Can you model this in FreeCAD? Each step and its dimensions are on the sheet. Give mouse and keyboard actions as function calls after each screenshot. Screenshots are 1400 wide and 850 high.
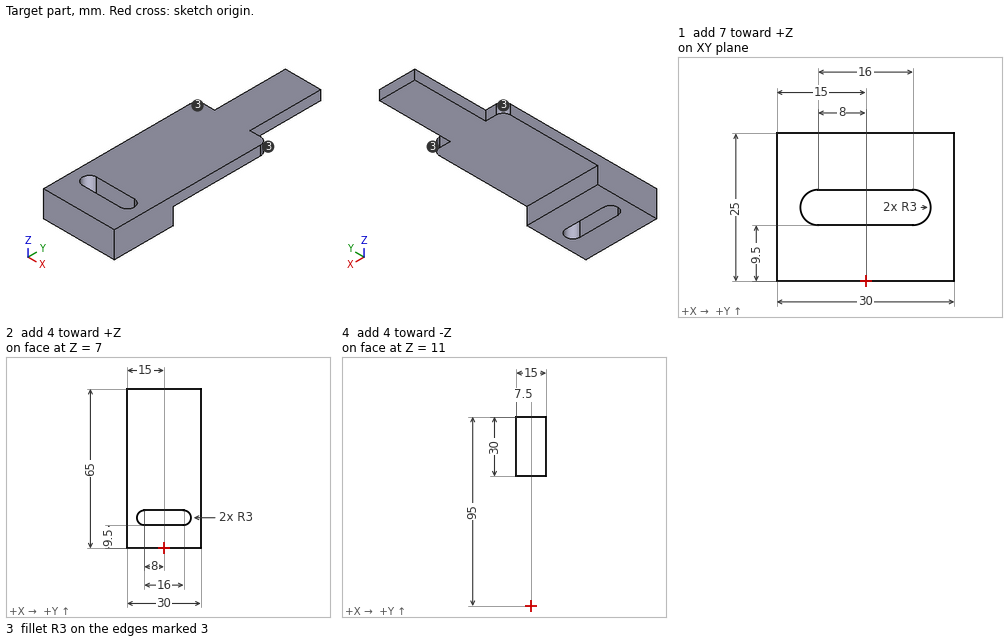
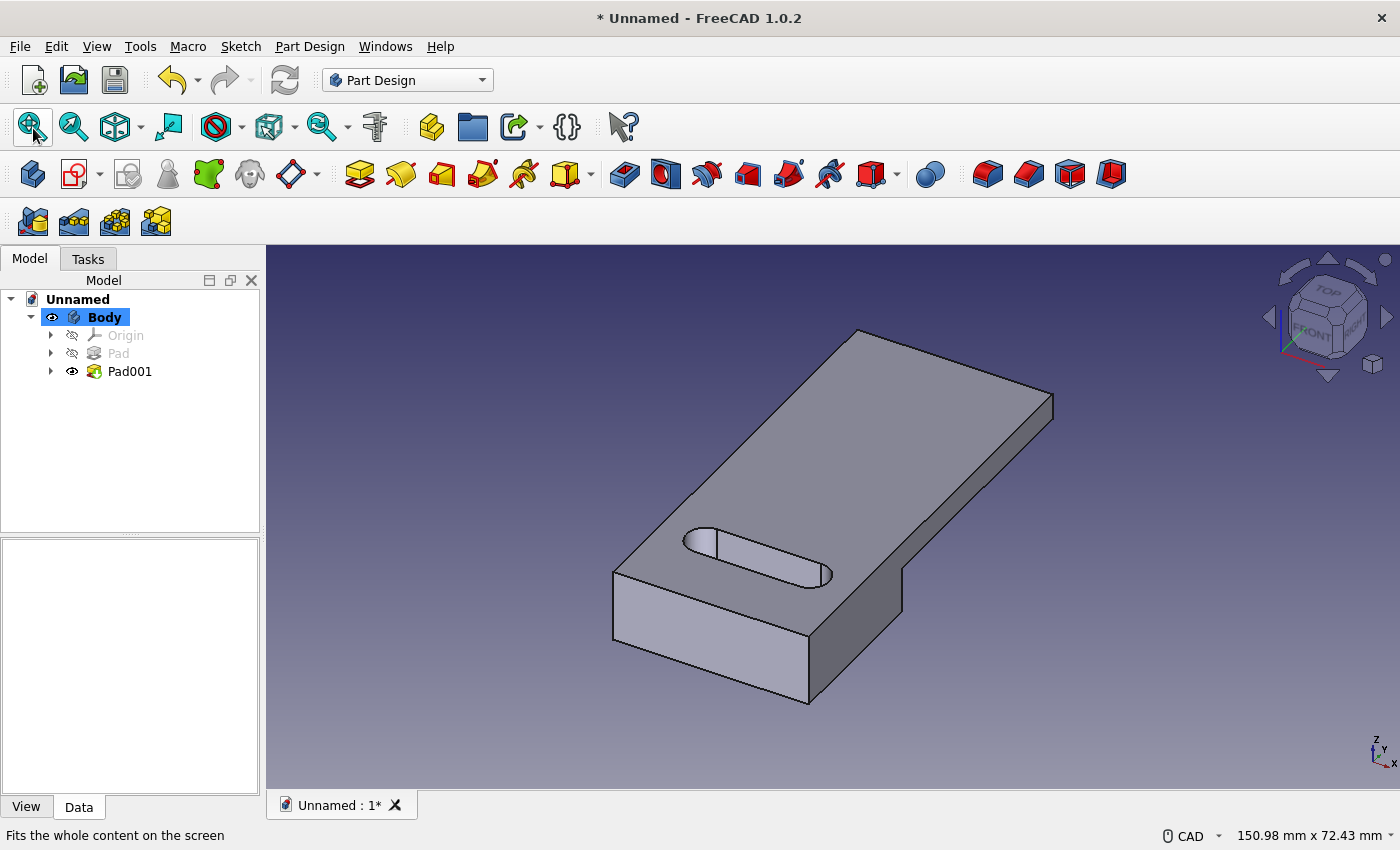
key(0)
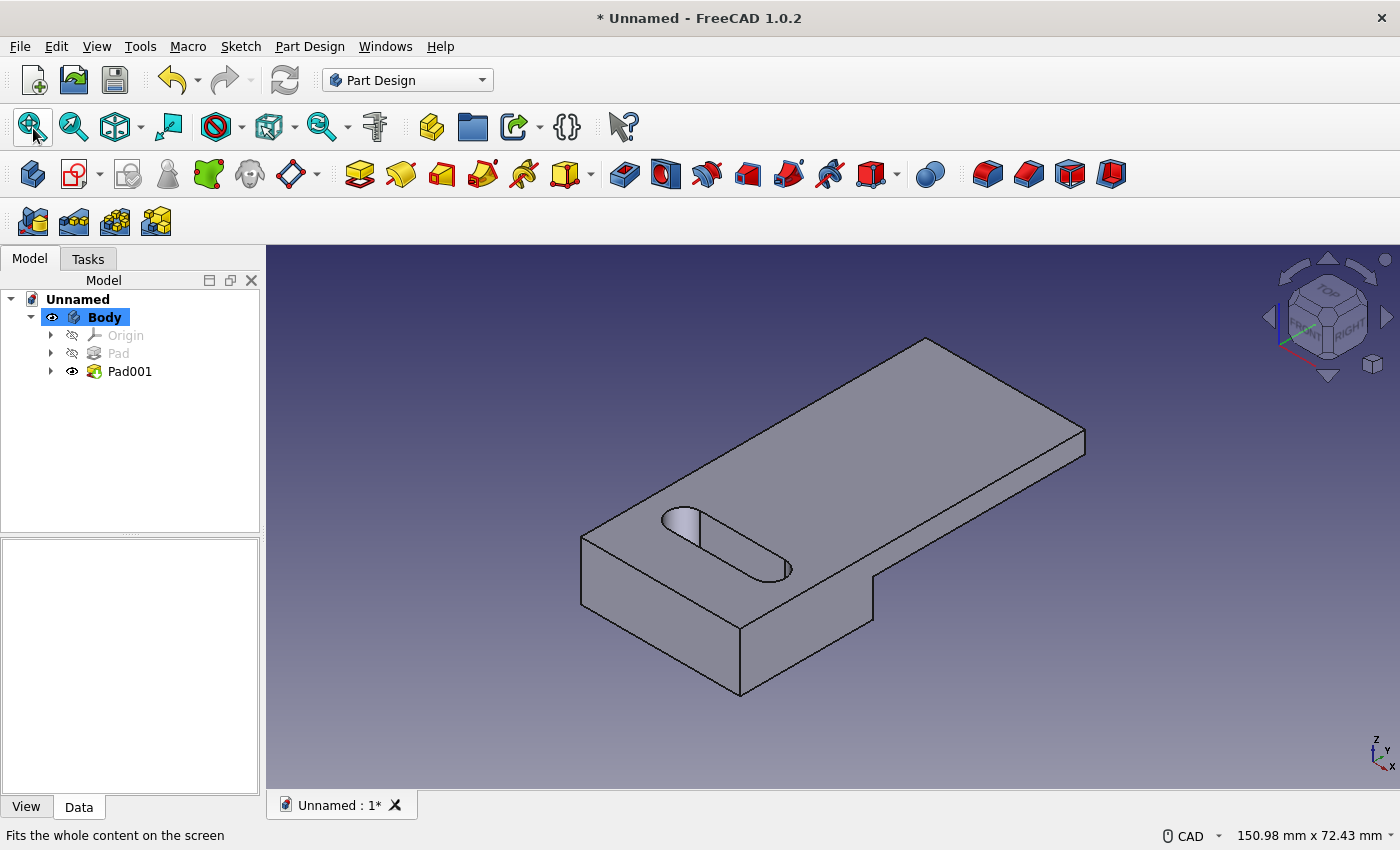
key(2)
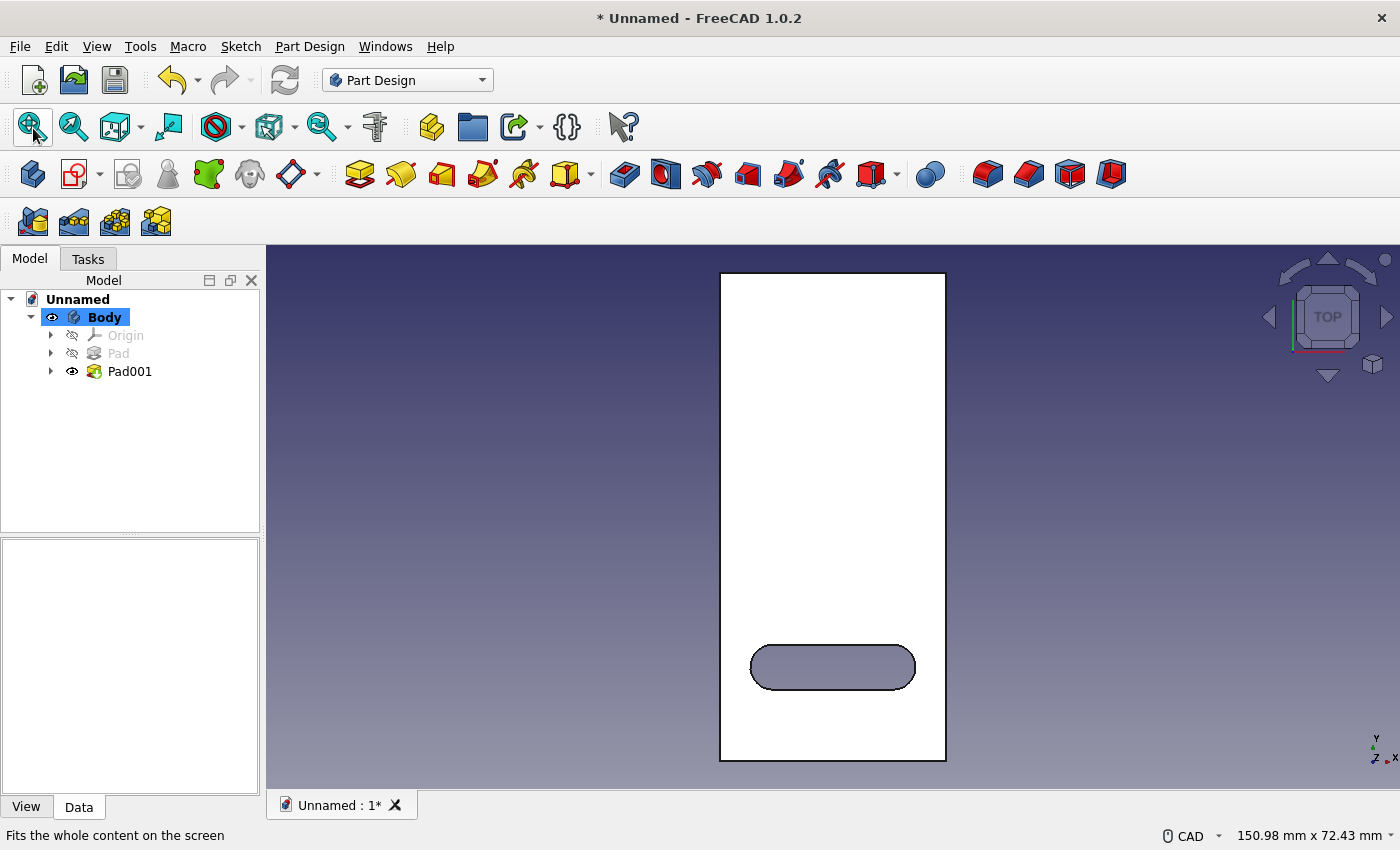
key(1)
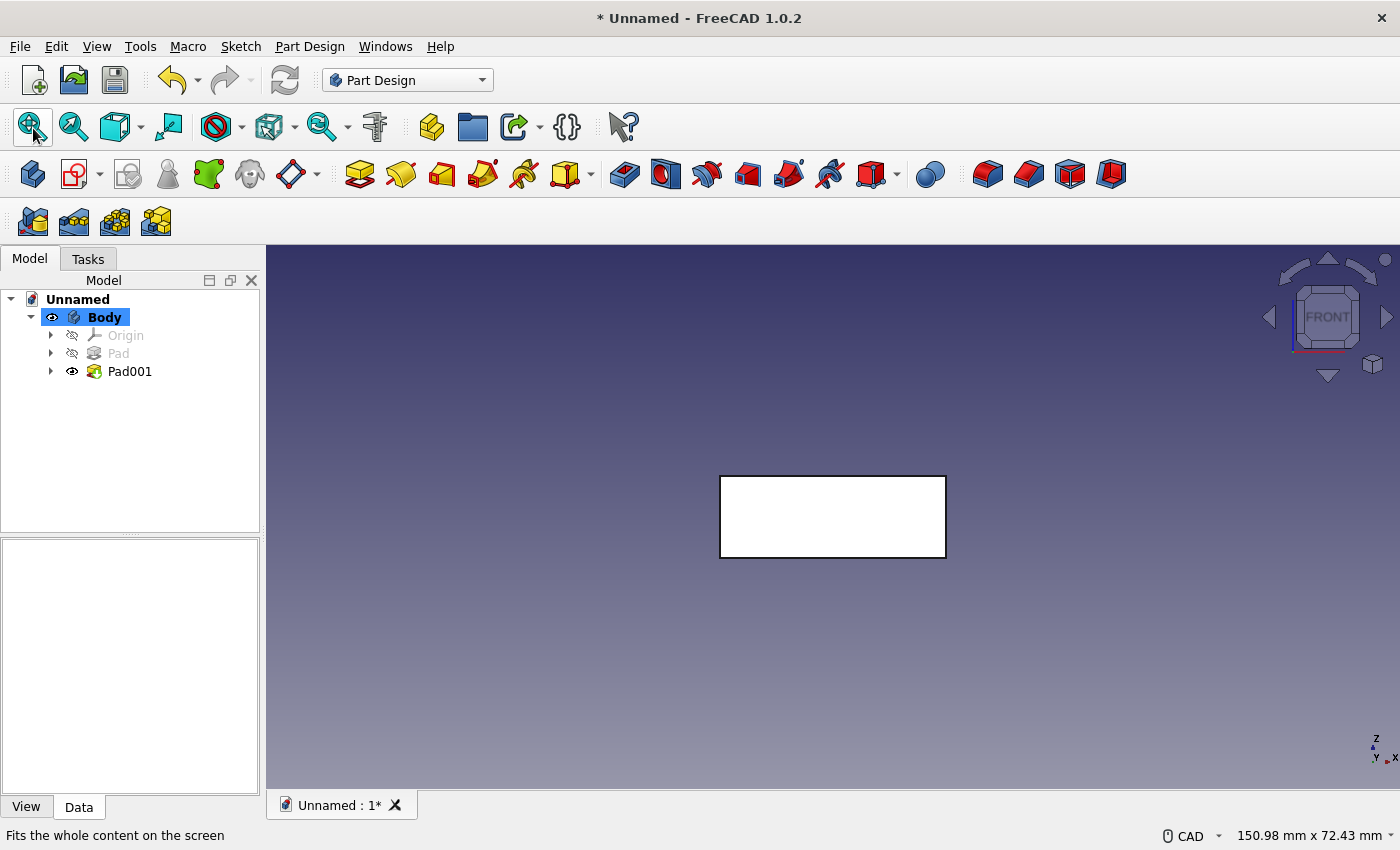
click(33, 128)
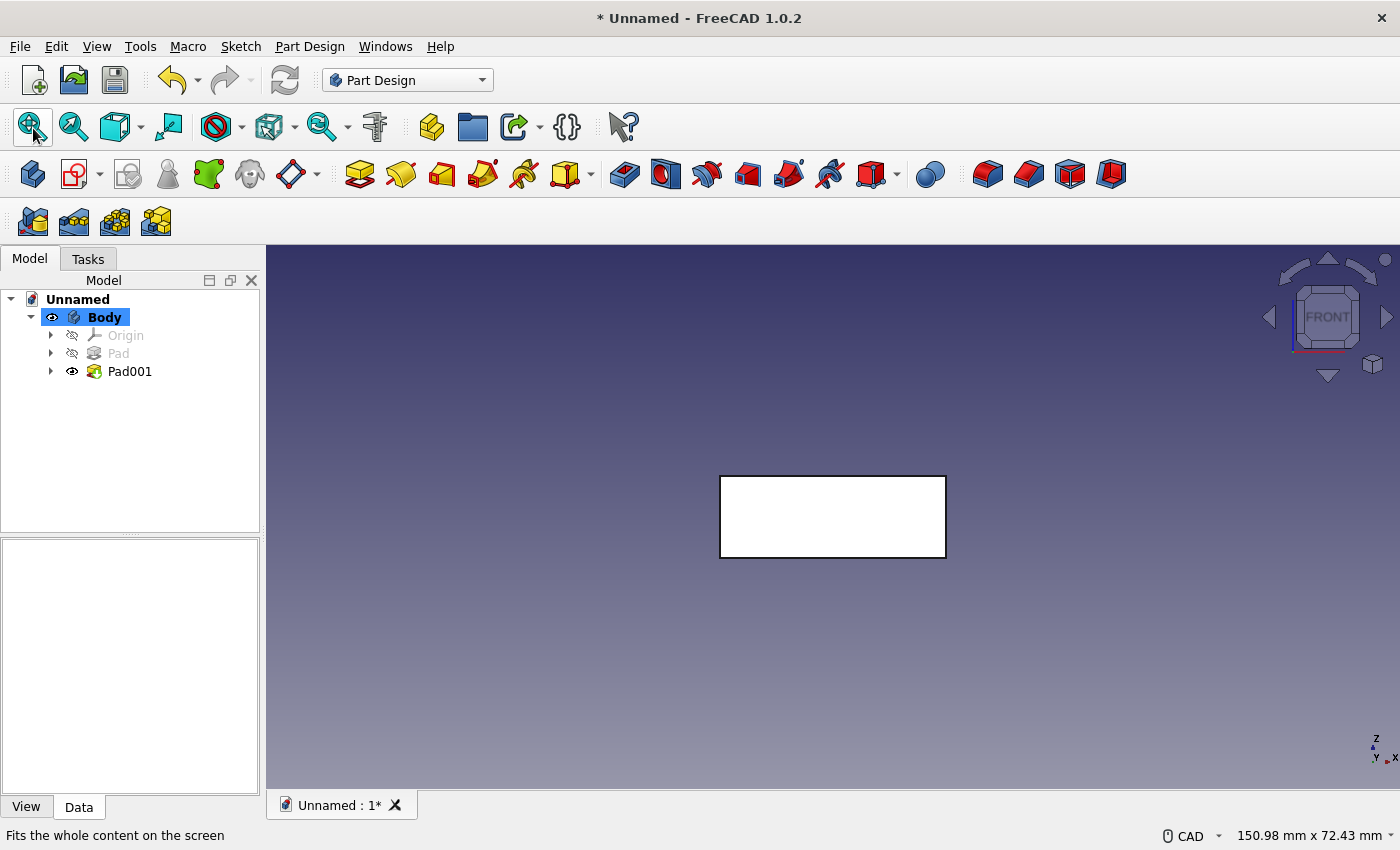
key(3)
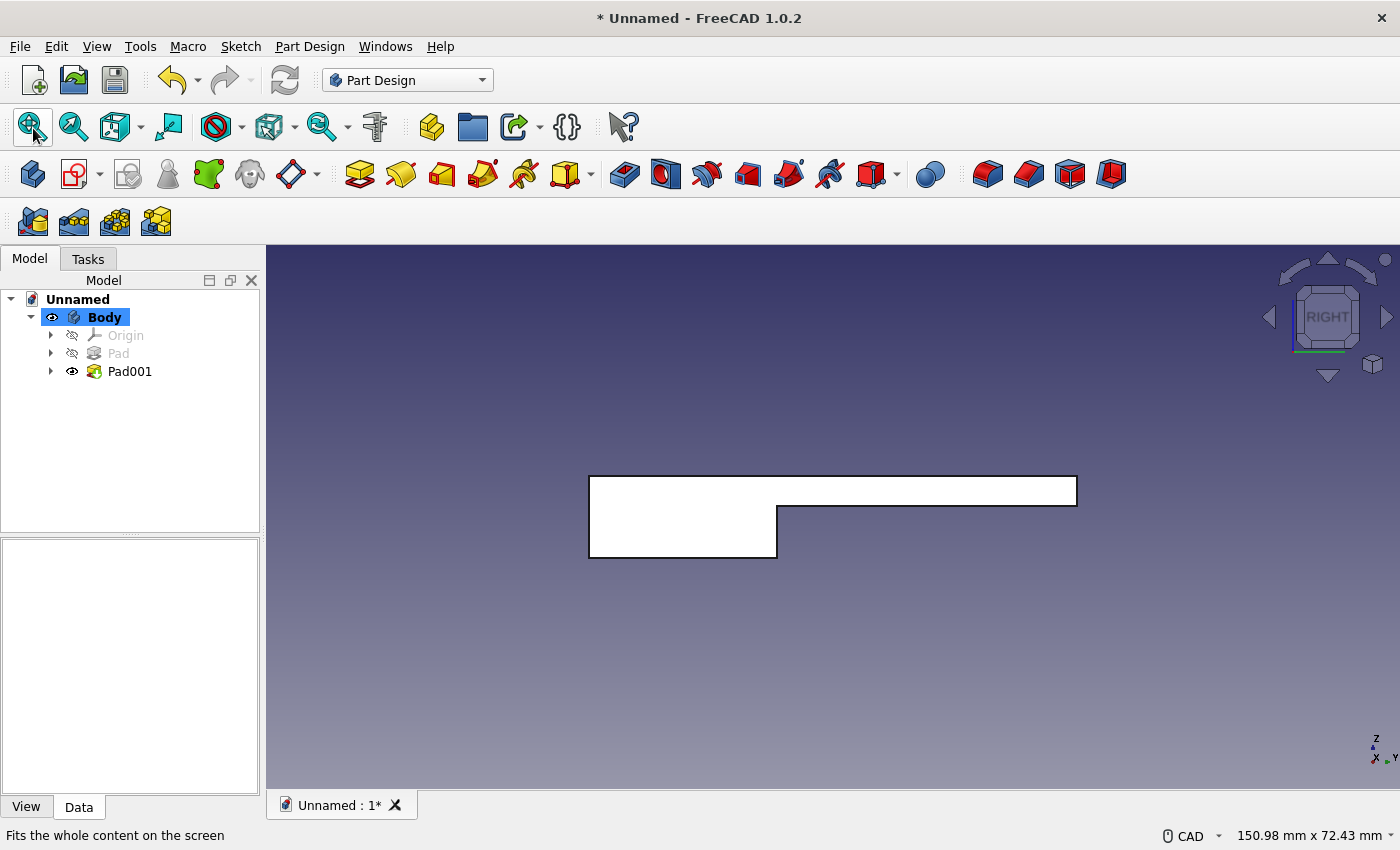
click(33, 128)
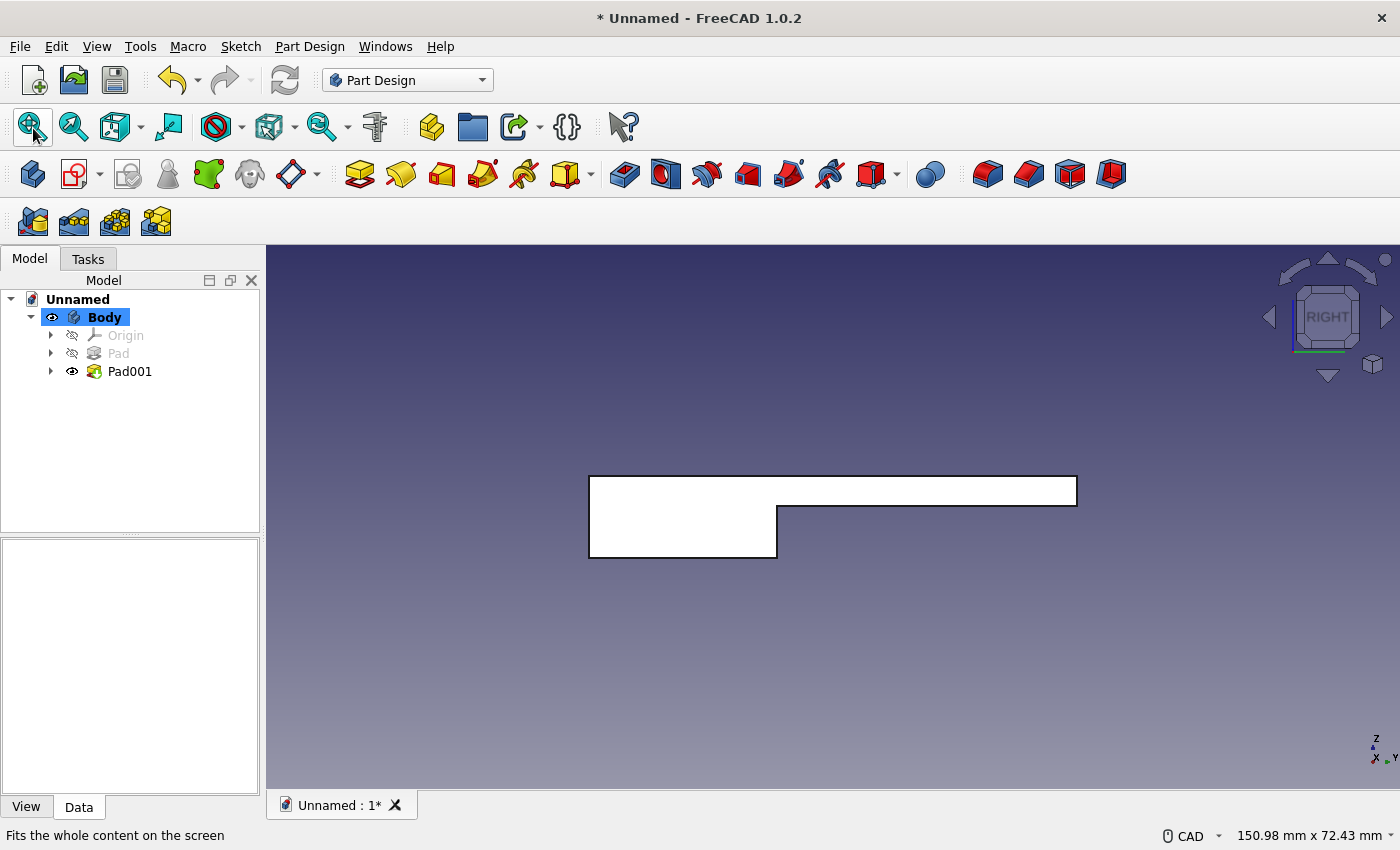
click(1077, 490)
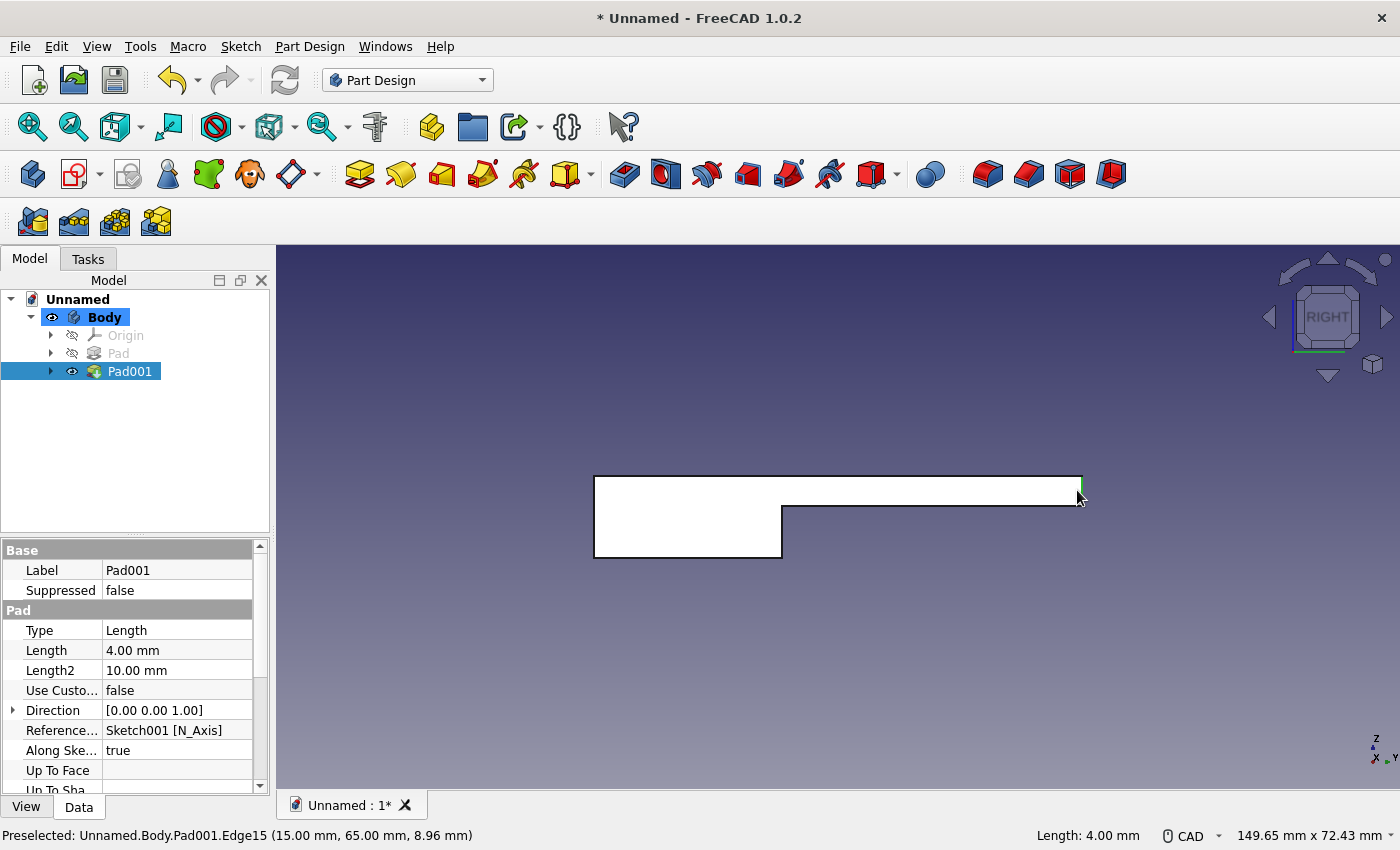
key(5)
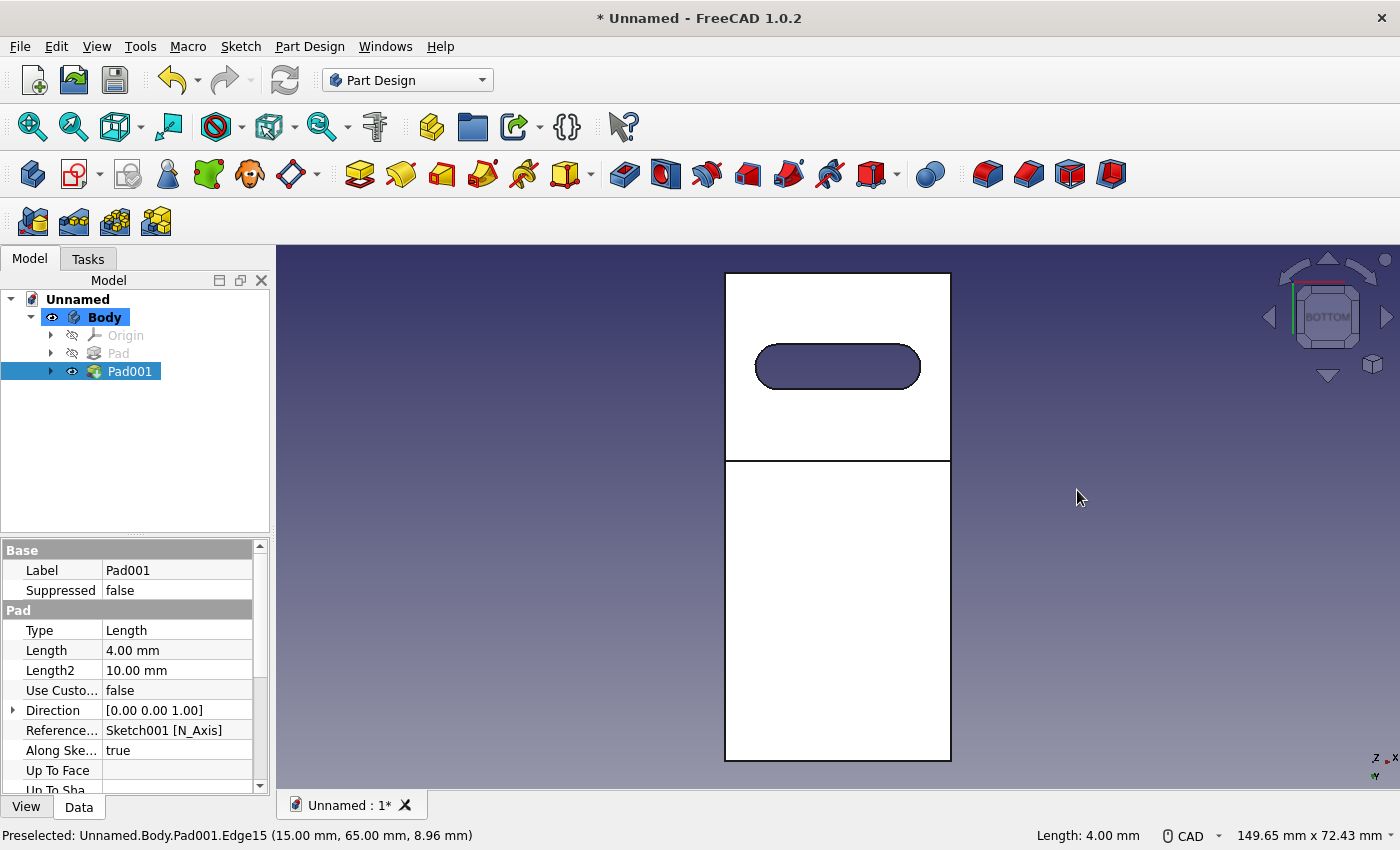
key(4)